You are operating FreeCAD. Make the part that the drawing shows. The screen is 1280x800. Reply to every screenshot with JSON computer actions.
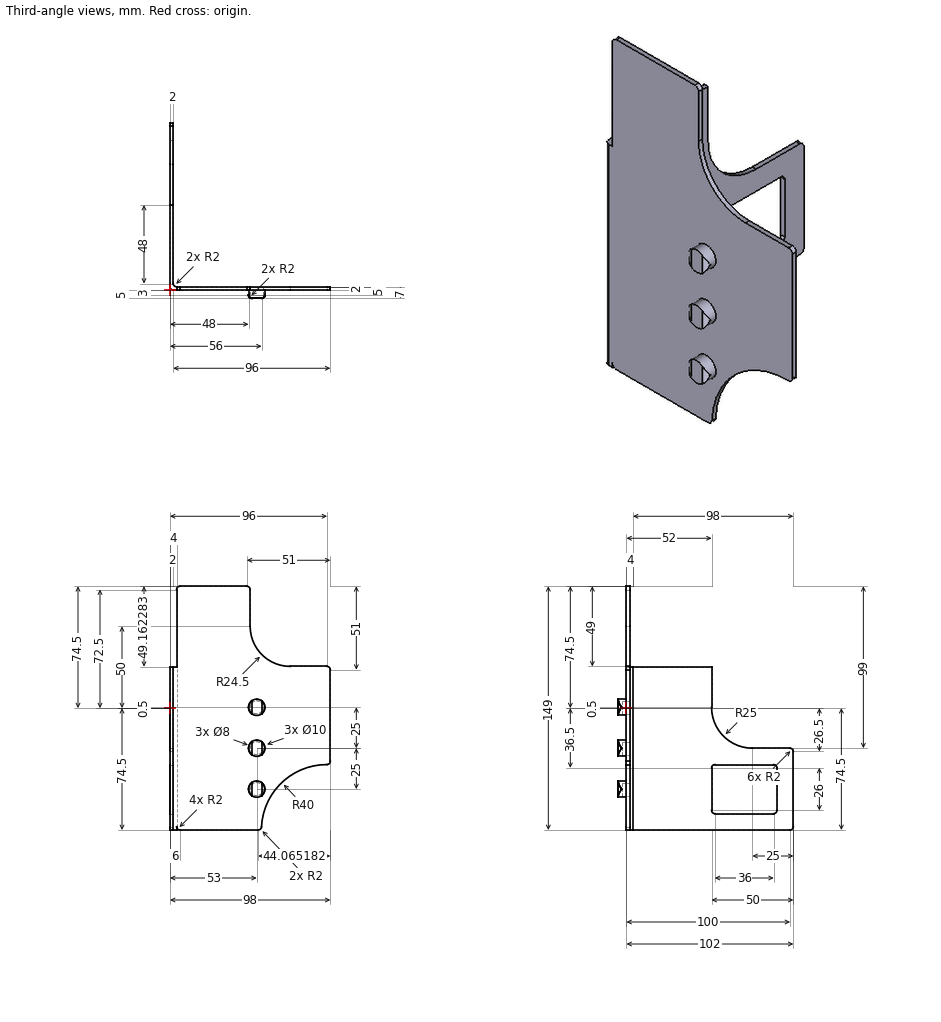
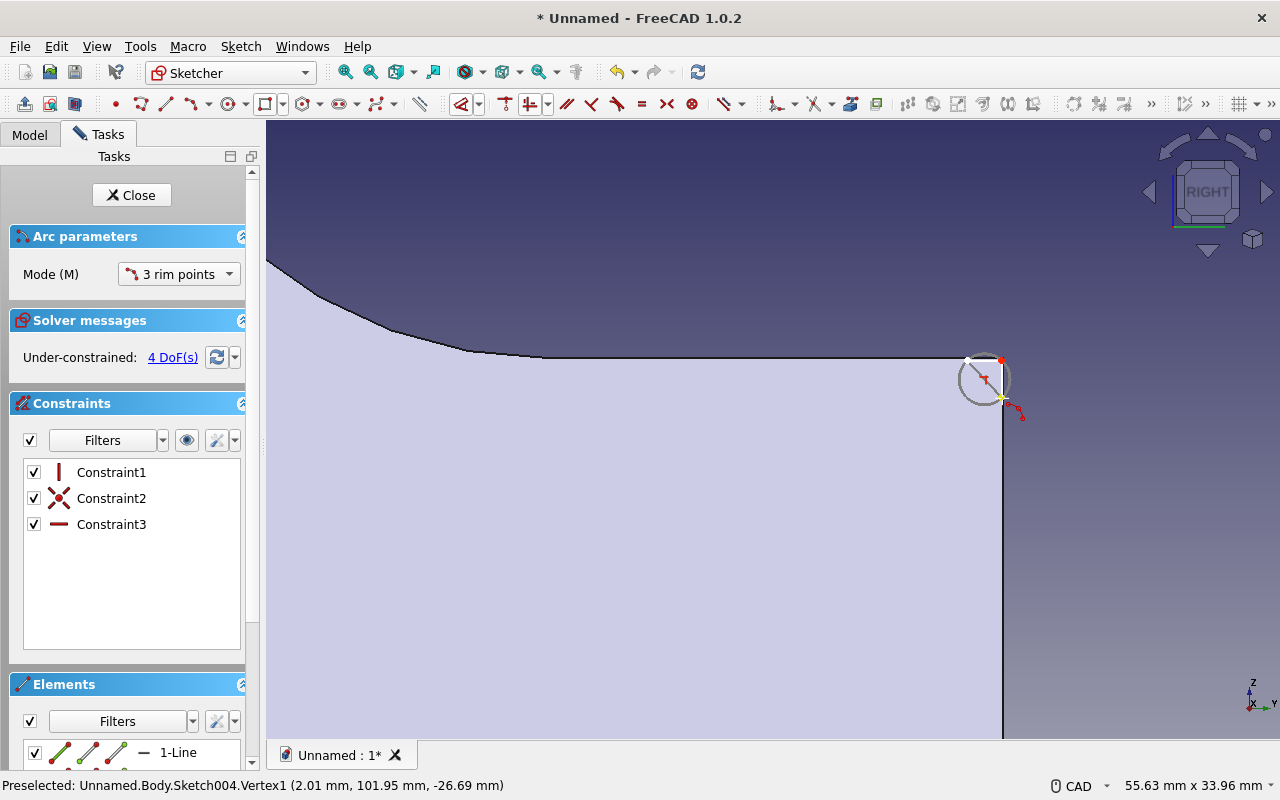
{"action": "scroll", "coordinate": [992, 369], "scroll_direction": "up", "scroll_amount": 2}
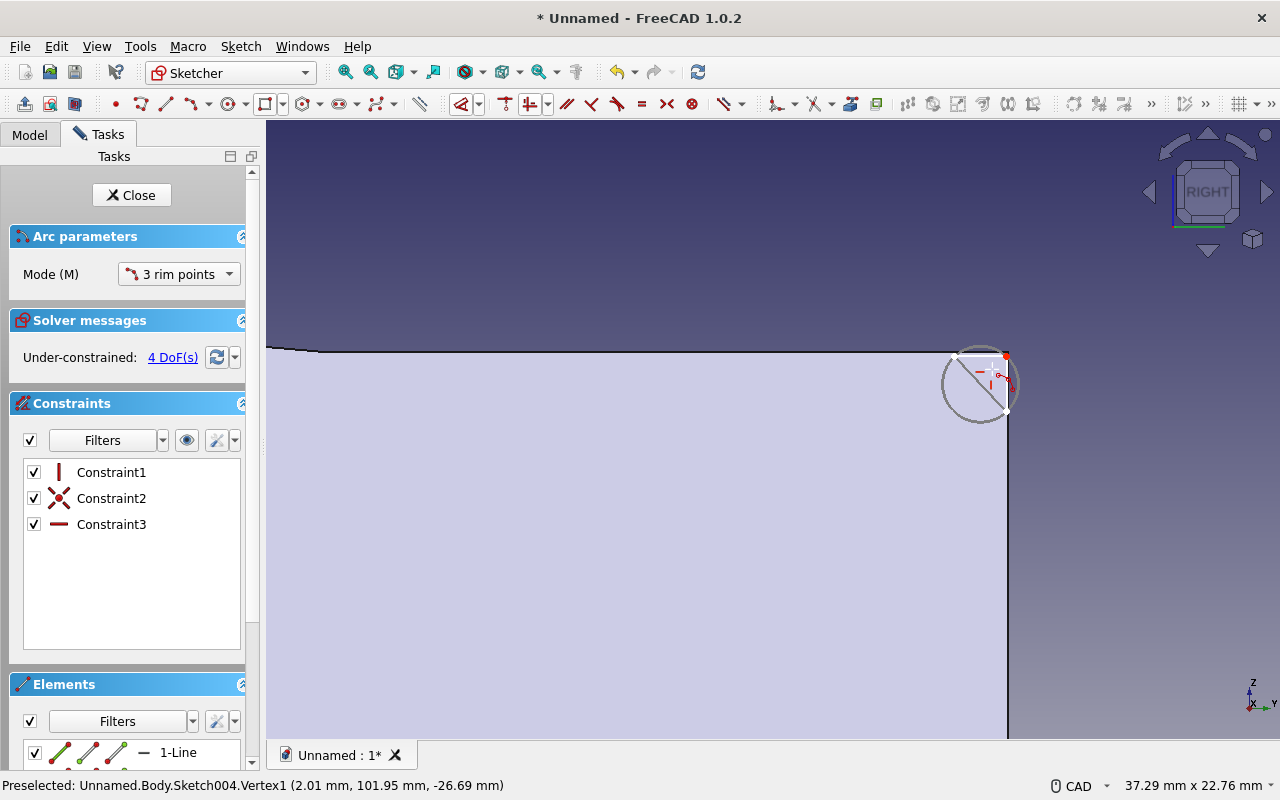
{"action": "left_click", "coordinate": [992, 368]}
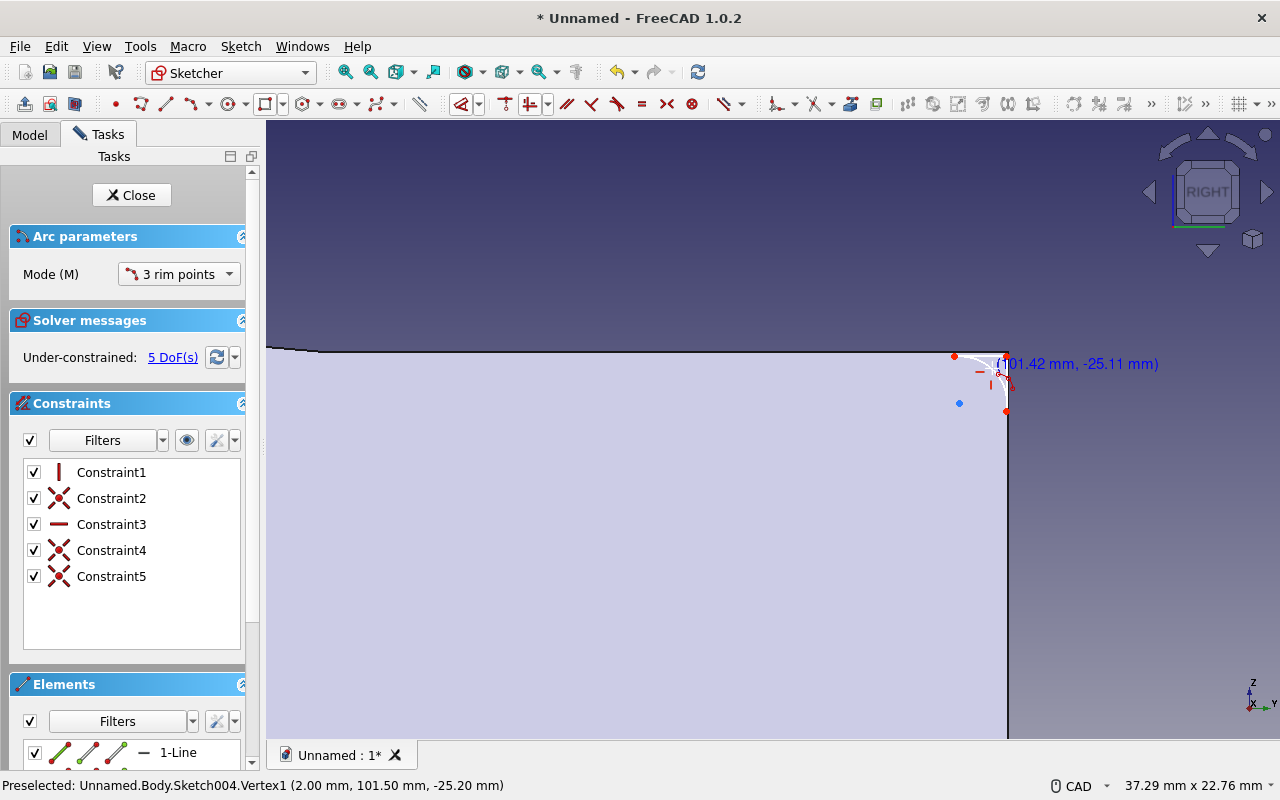
{"action": "key", "text": "g m"}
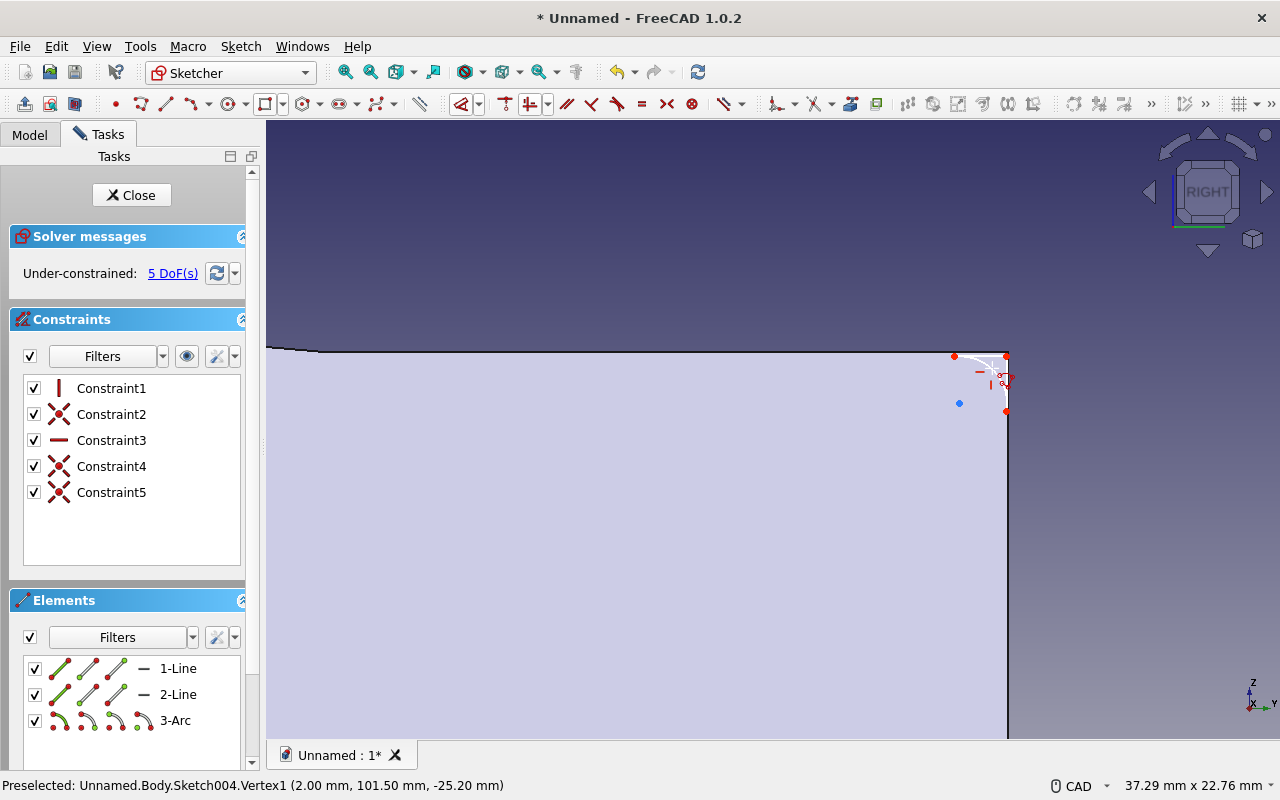
{"action": "scroll", "coordinate": [979, 361], "scroll_direction": "down", "scroll_amount": 8}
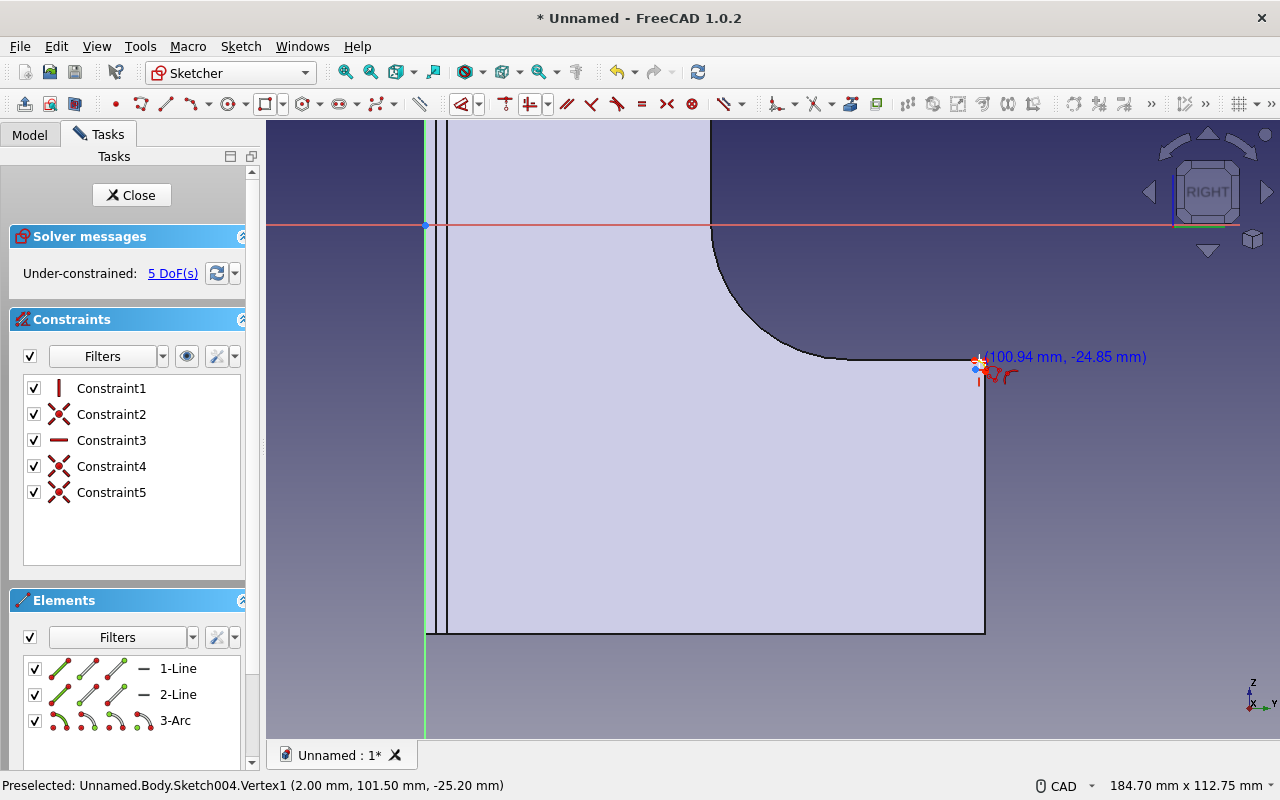
{"action": "left_click", "coordinate": [974, 634]}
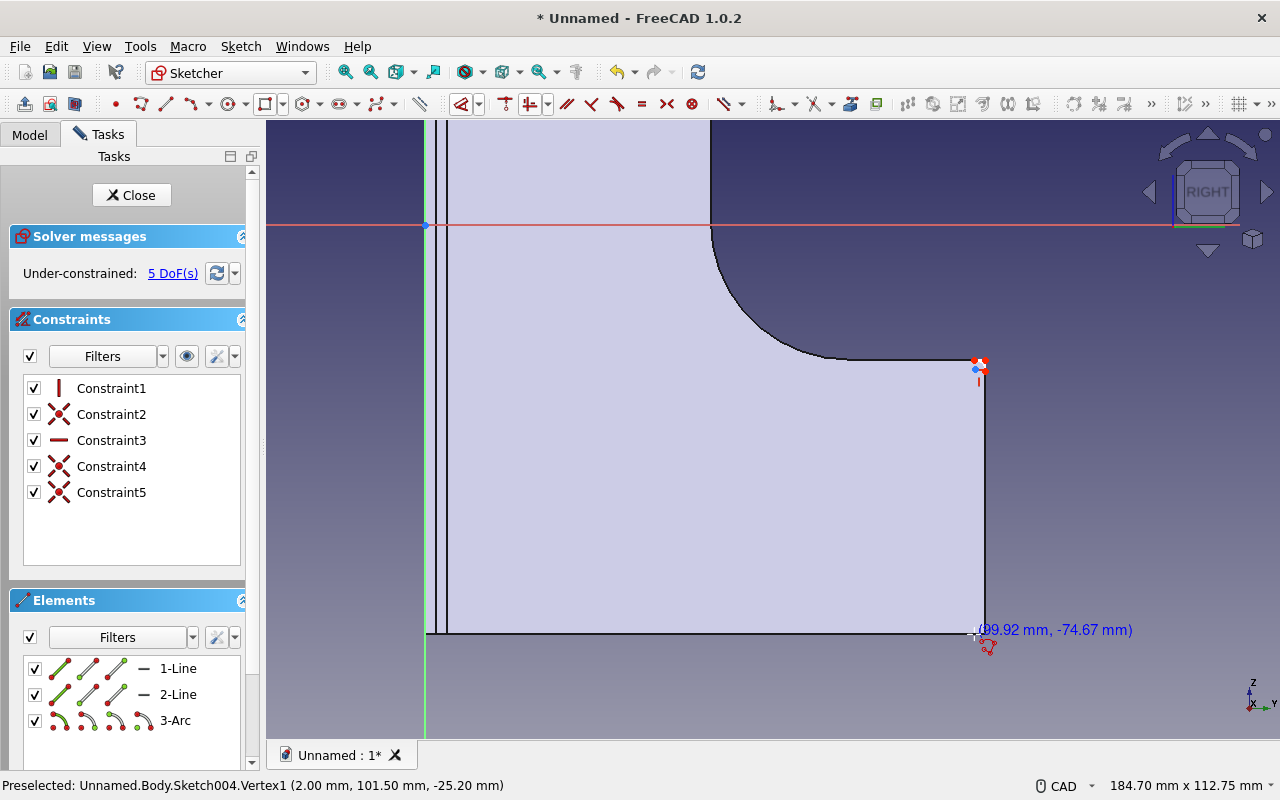
{"action": "scroll", "coordinate": [985, 634], "scroll_direction": "up", "scroll_amount": 2}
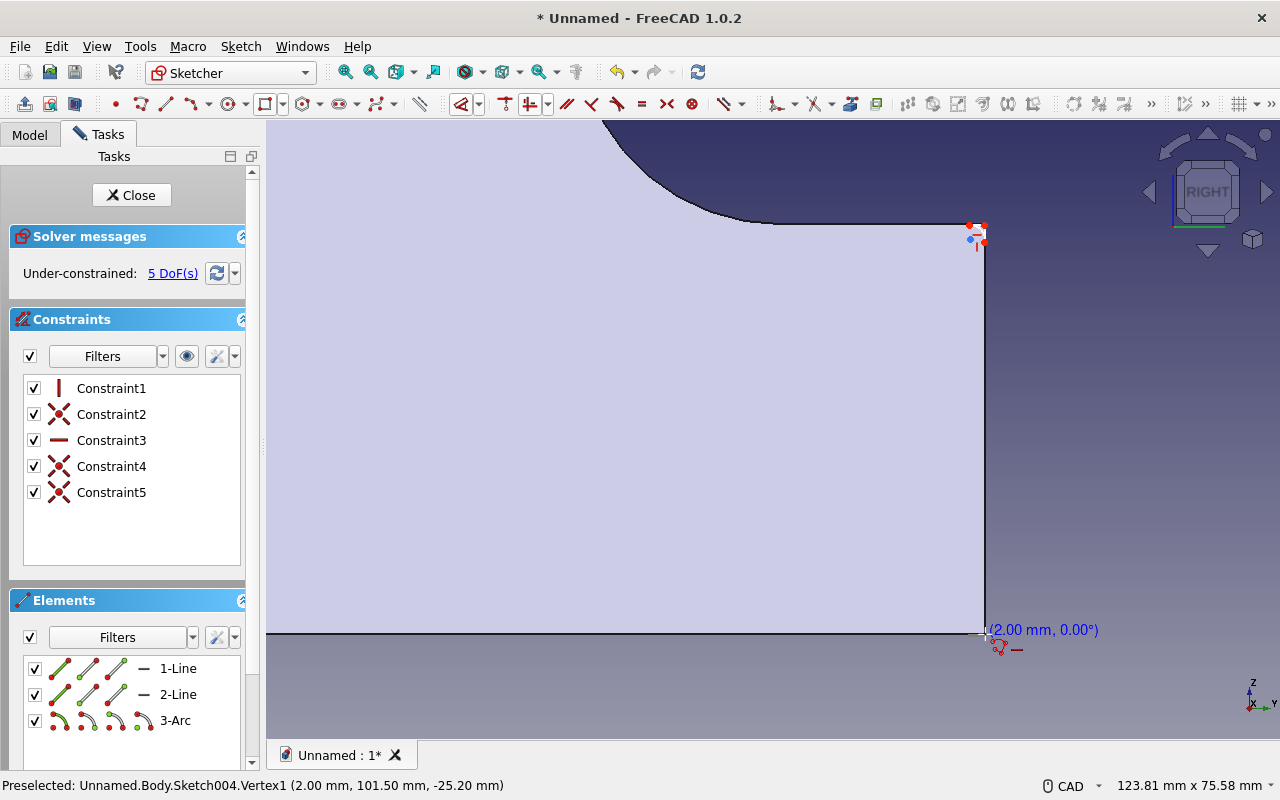
{"action": "left_click", "coordinate": [985, 634]}
{"action": "left_click", "coordinate": [985, 617]}
{"action": "right_click", "coordinate": [985, 617]}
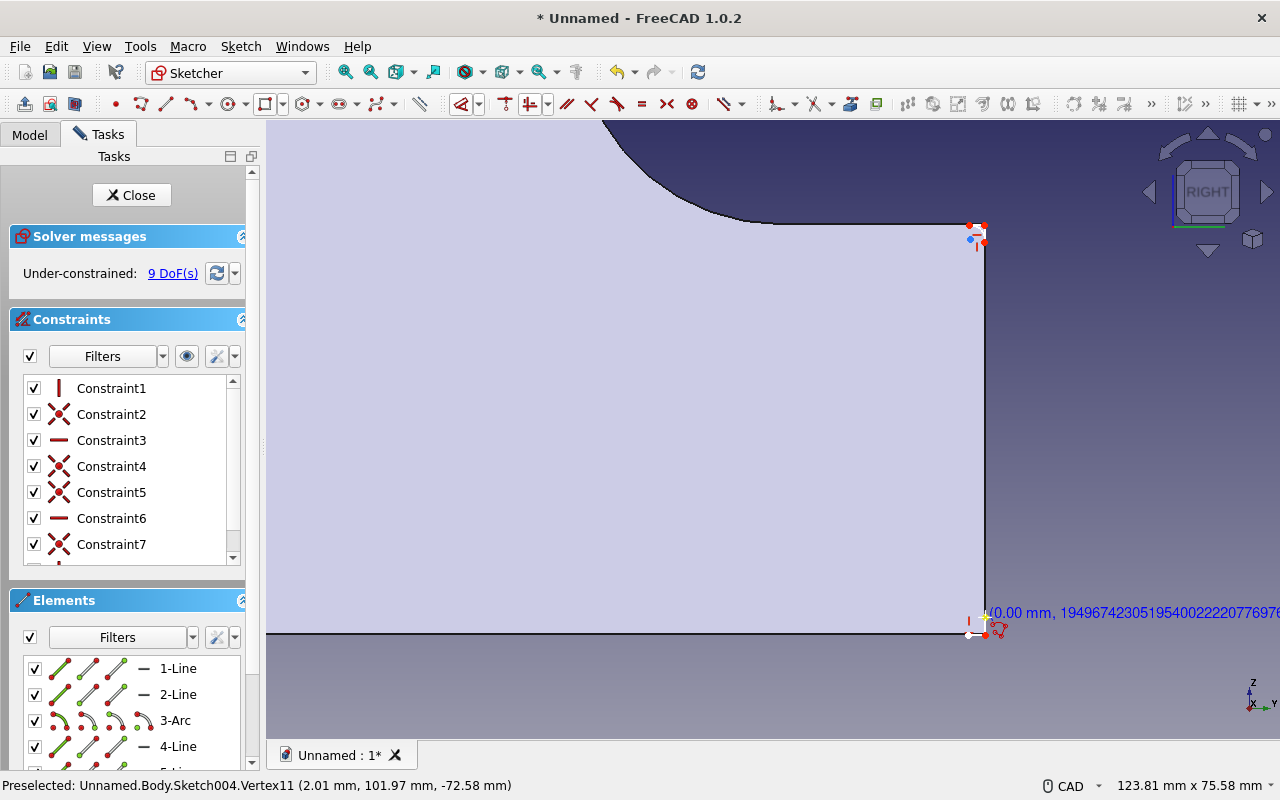
{"action": "left_click", "coordinate": [190, 104]}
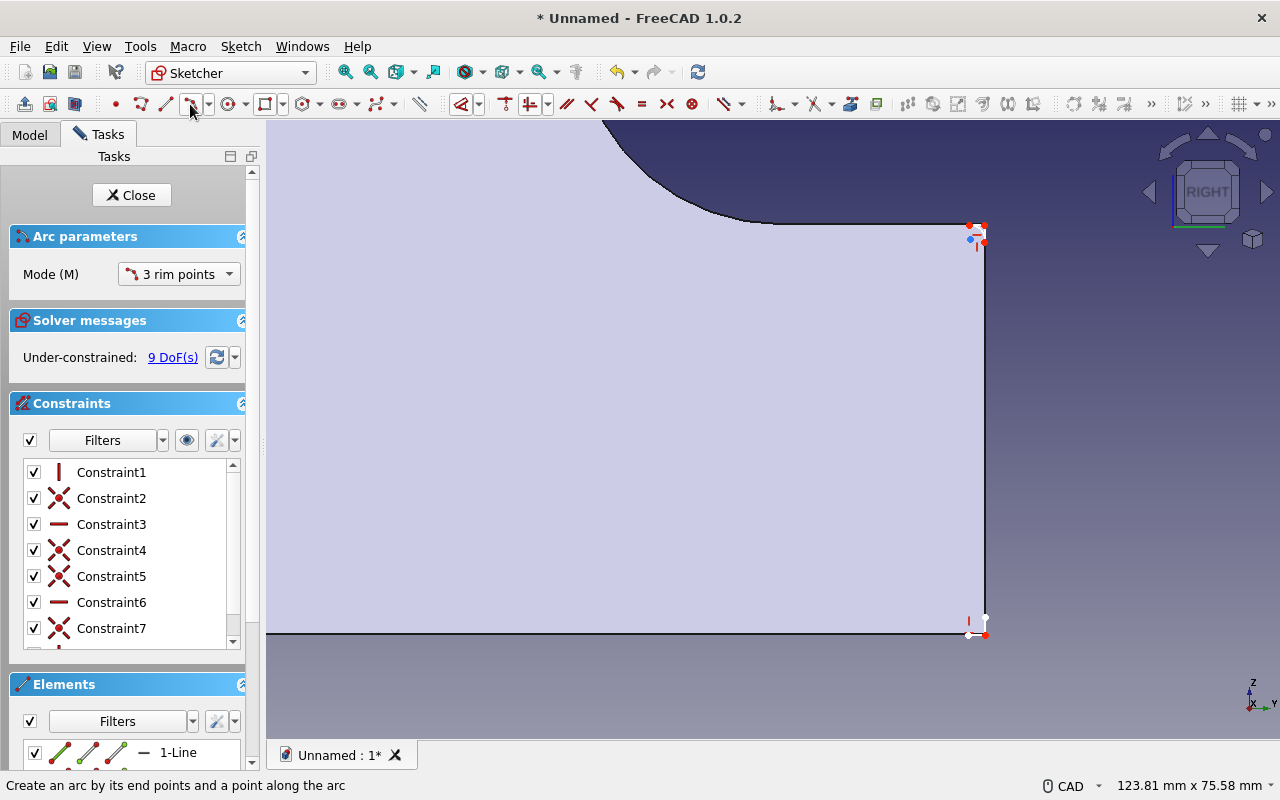
{"action": "scroll", "coordinate": [985, 617], "scroll_direction": "up", "scroll_amount": 4}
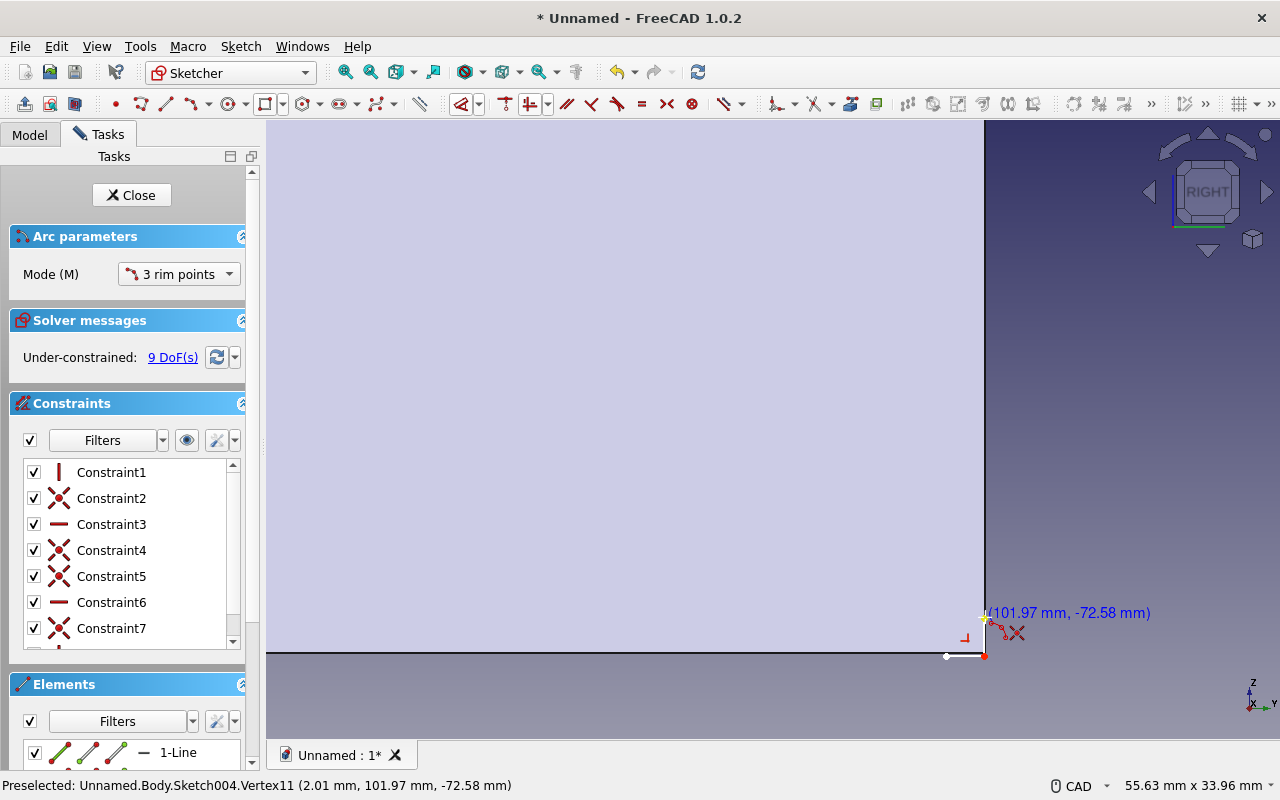
{"action": "left_click", "coordinate": [984, 618]}
{"action": "left_click", "coordinate": [947, 656]}